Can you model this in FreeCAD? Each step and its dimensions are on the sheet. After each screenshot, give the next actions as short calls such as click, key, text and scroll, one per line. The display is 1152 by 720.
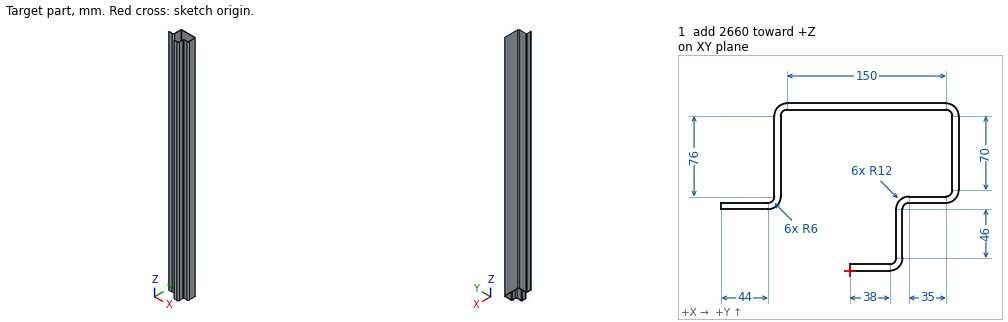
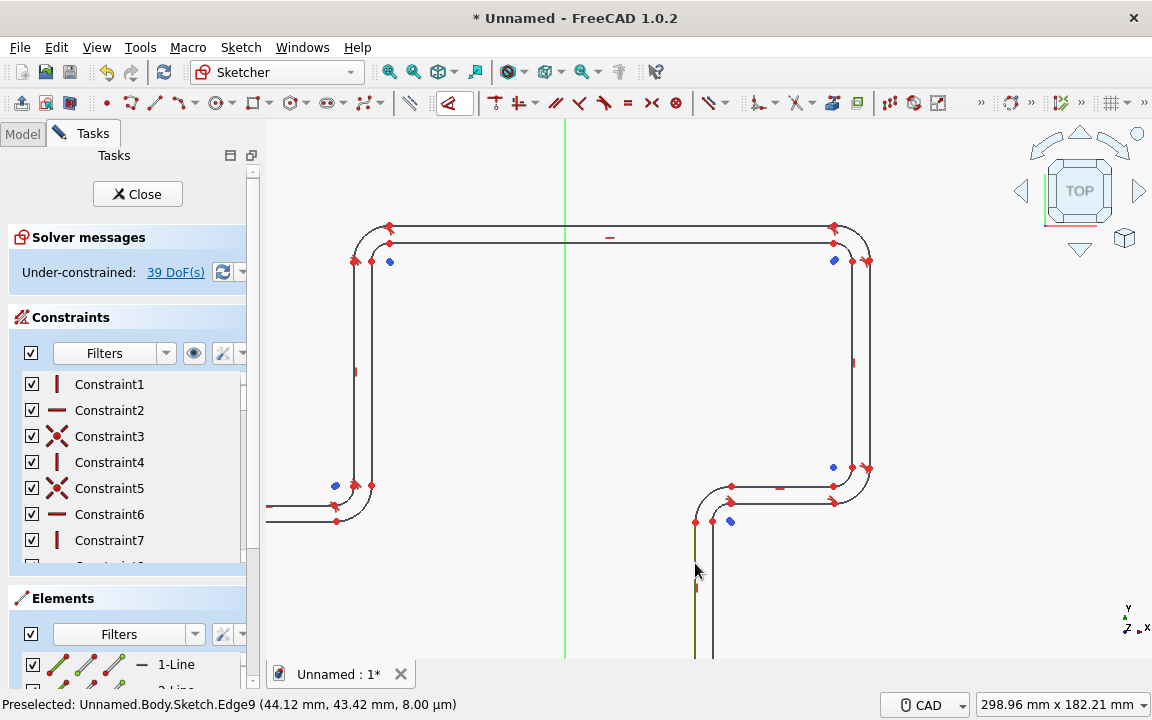
click(715, 491)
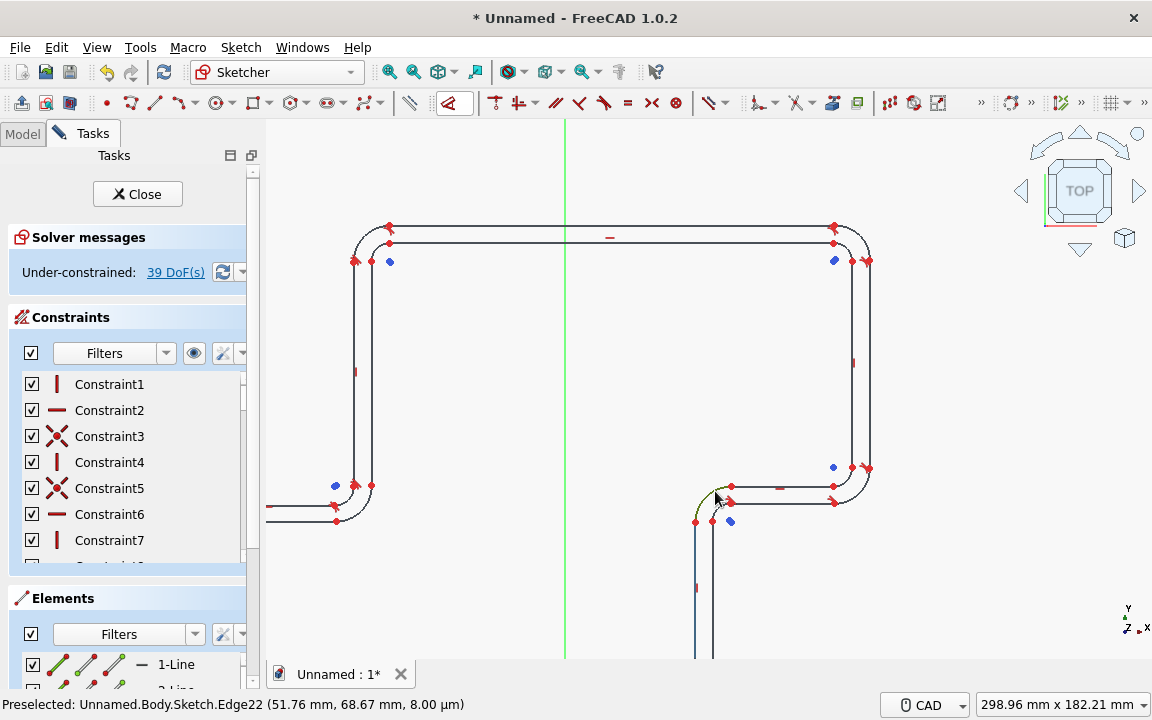
key(t)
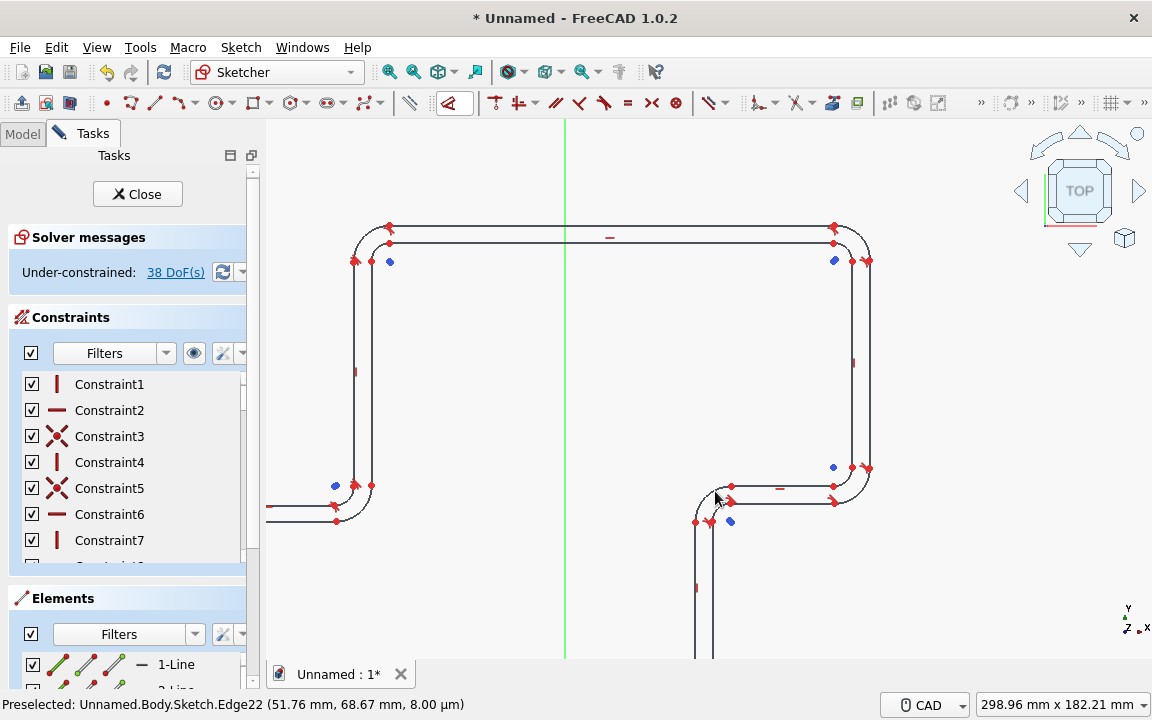
click(695, 563)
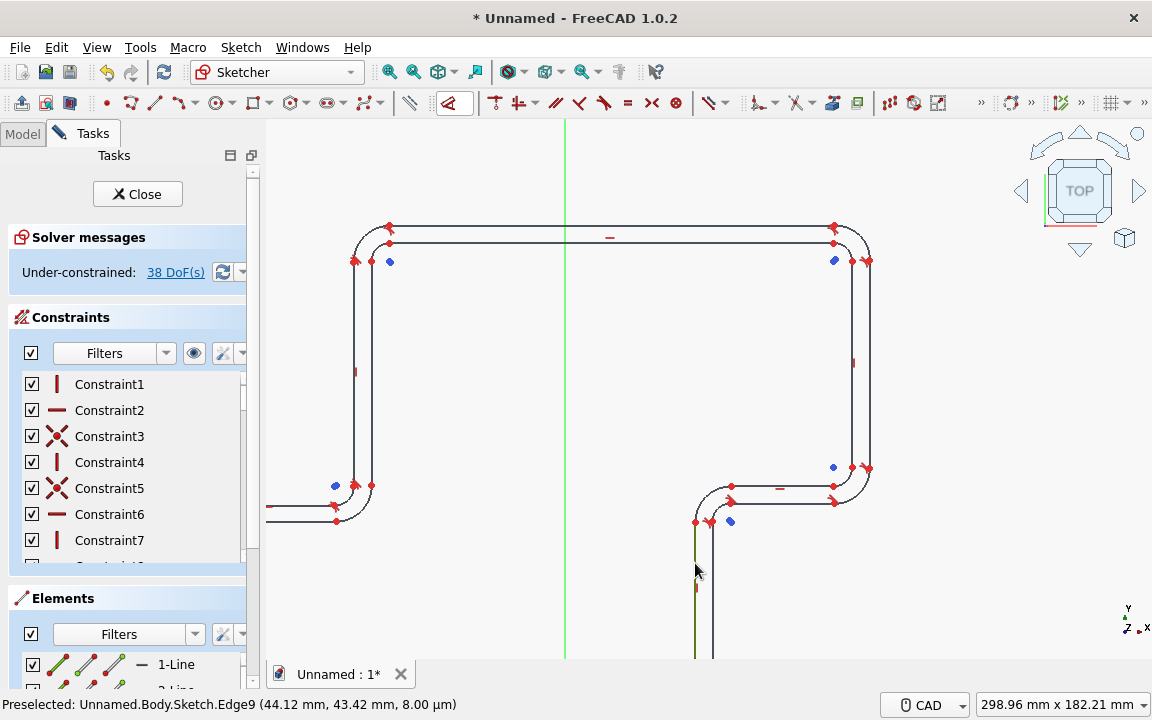
scroll(849, 248, down, 2)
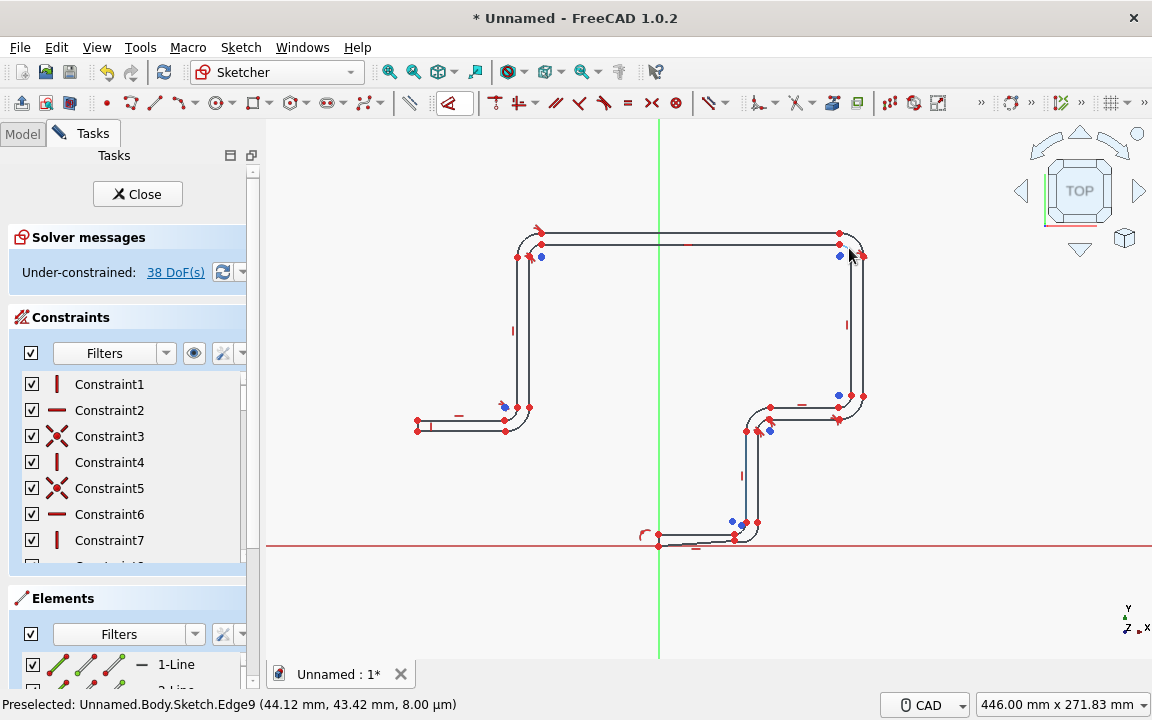
scroll(742, 531, up, 3)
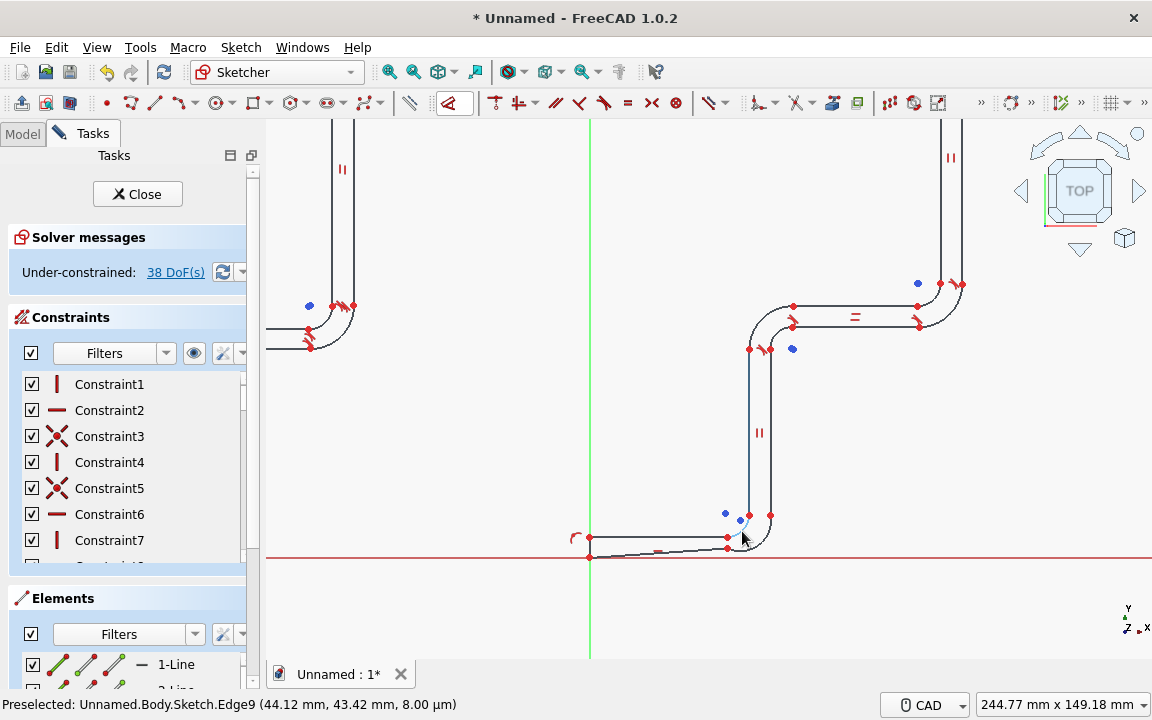
click(742, 530)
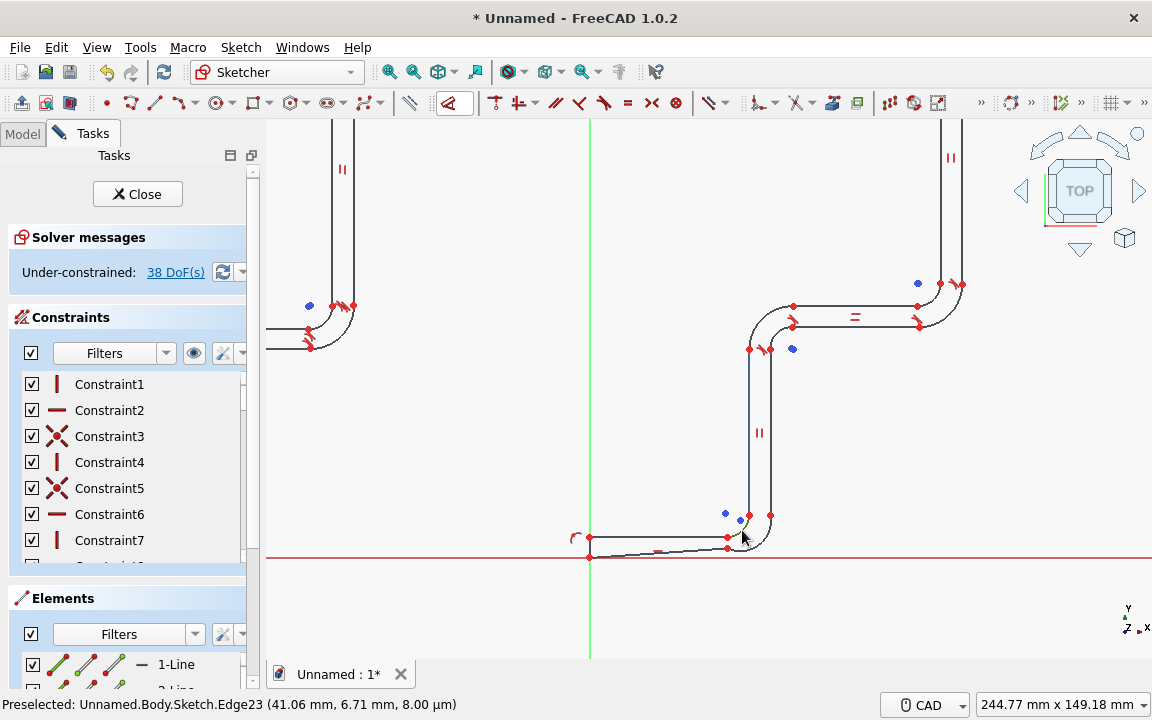
click(604, 104)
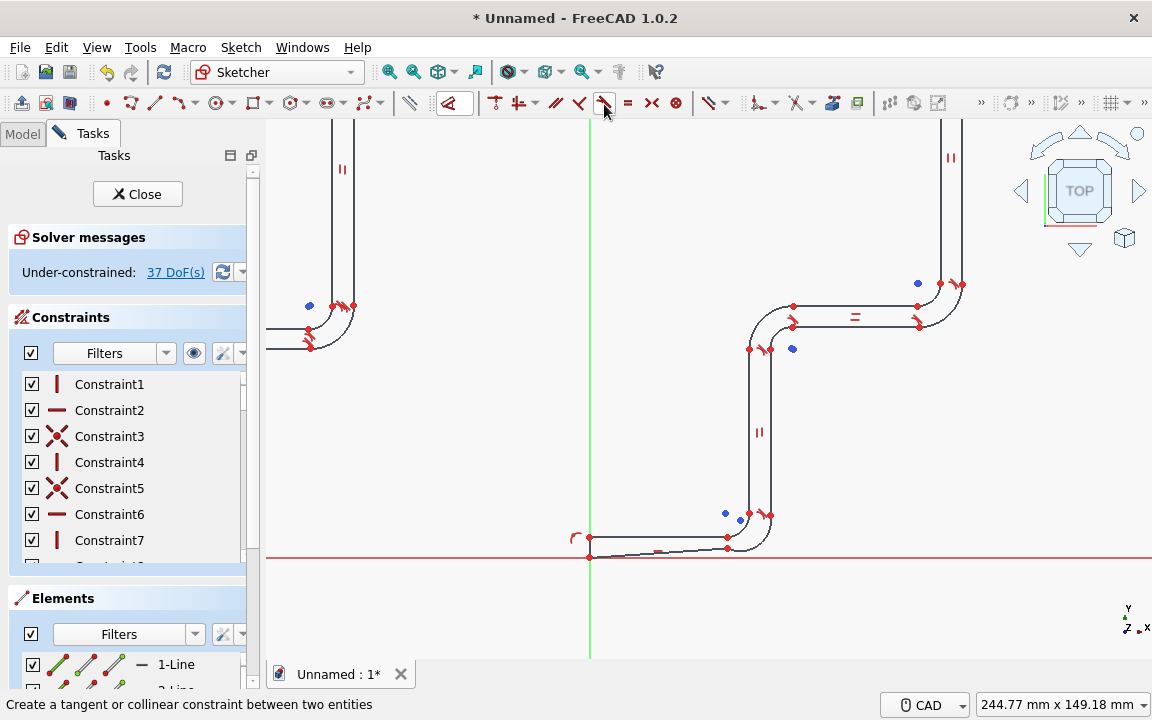
click(686, 537)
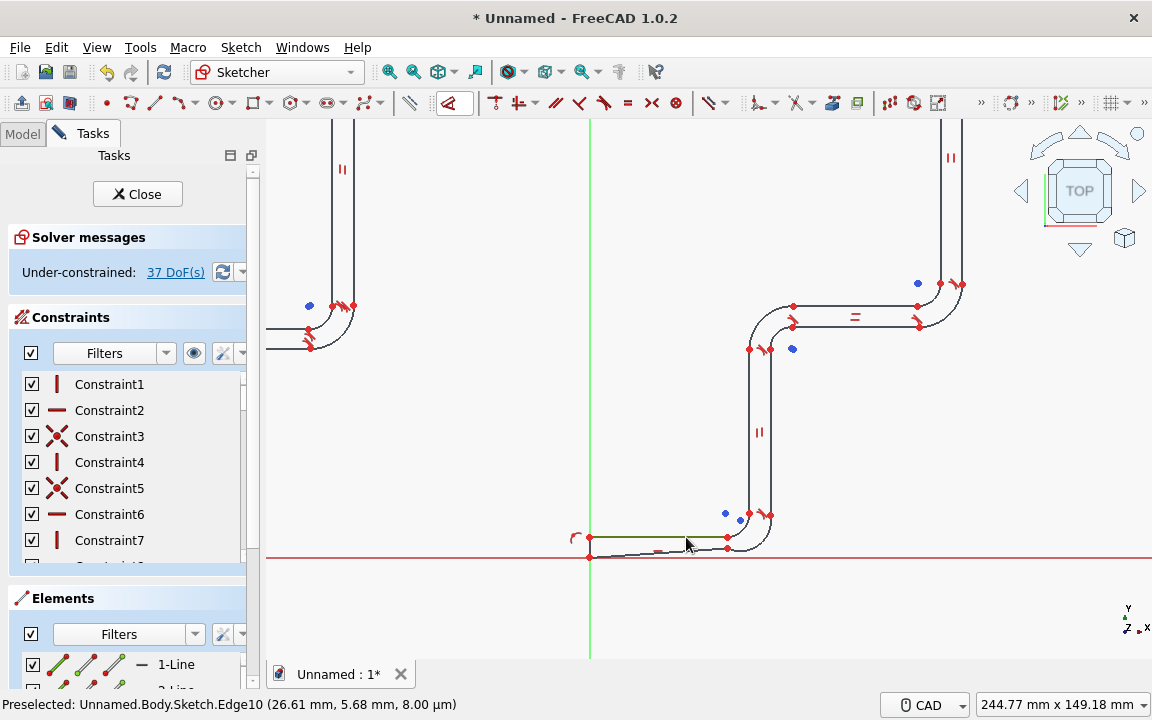
scroll(738, 534, up, 2)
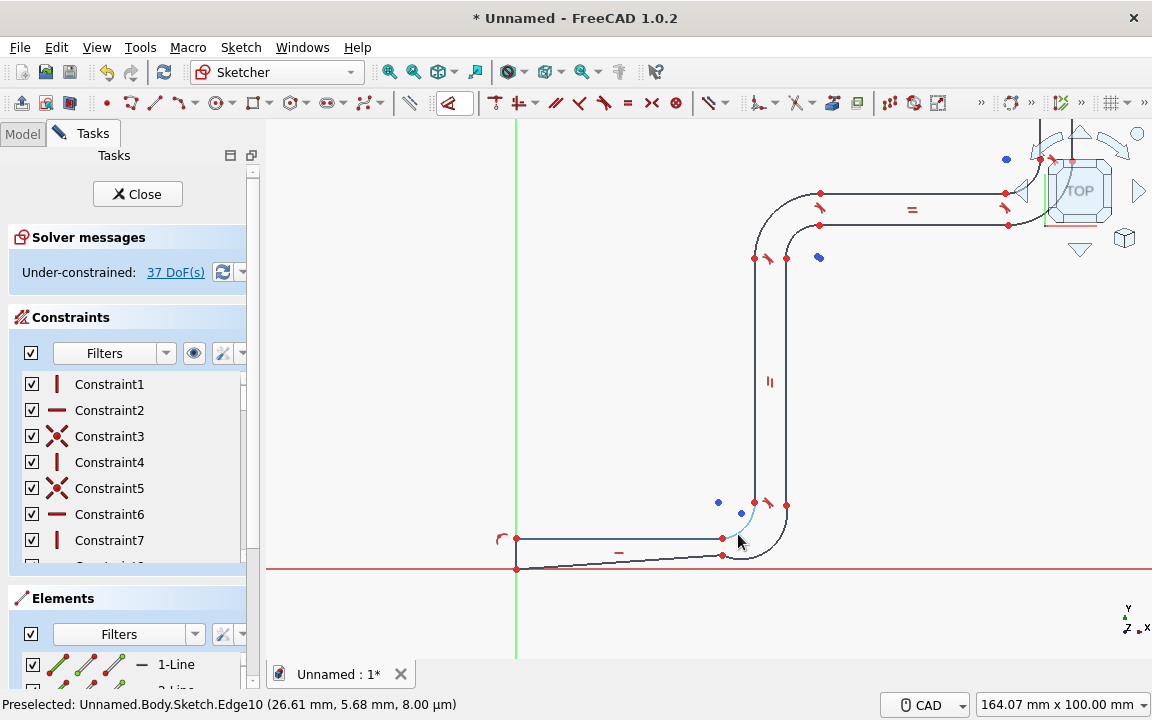
click(737, 534)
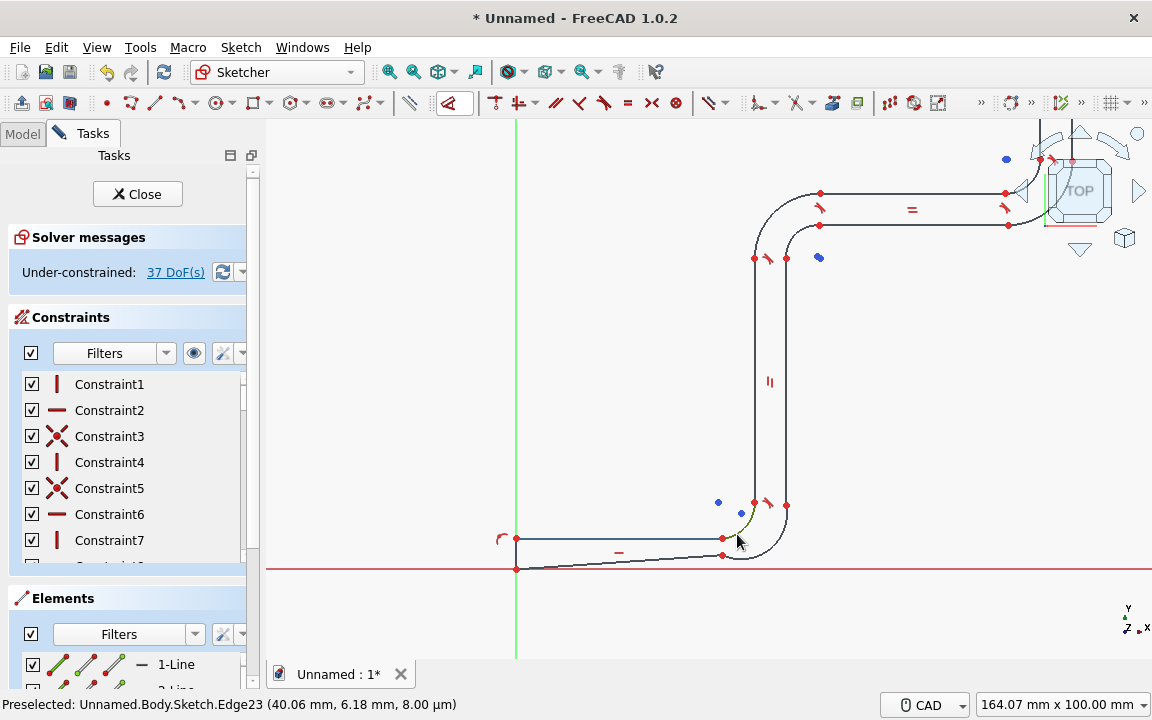
key(t)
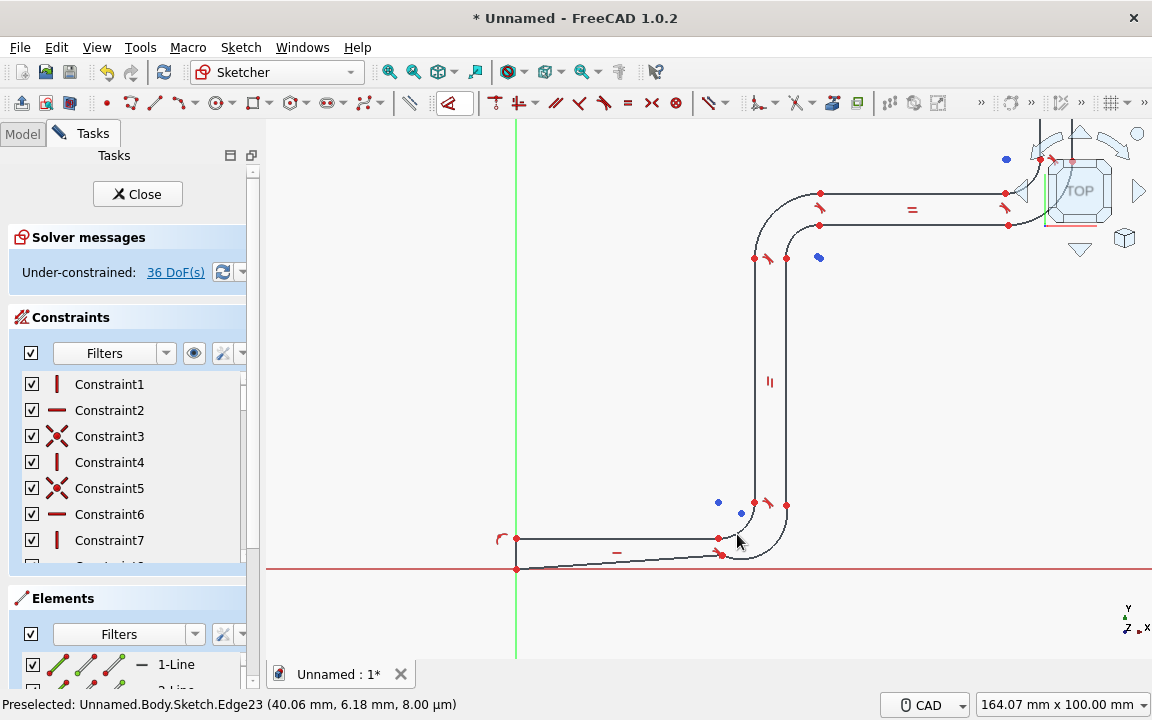
scroll(661, 559, up, 2)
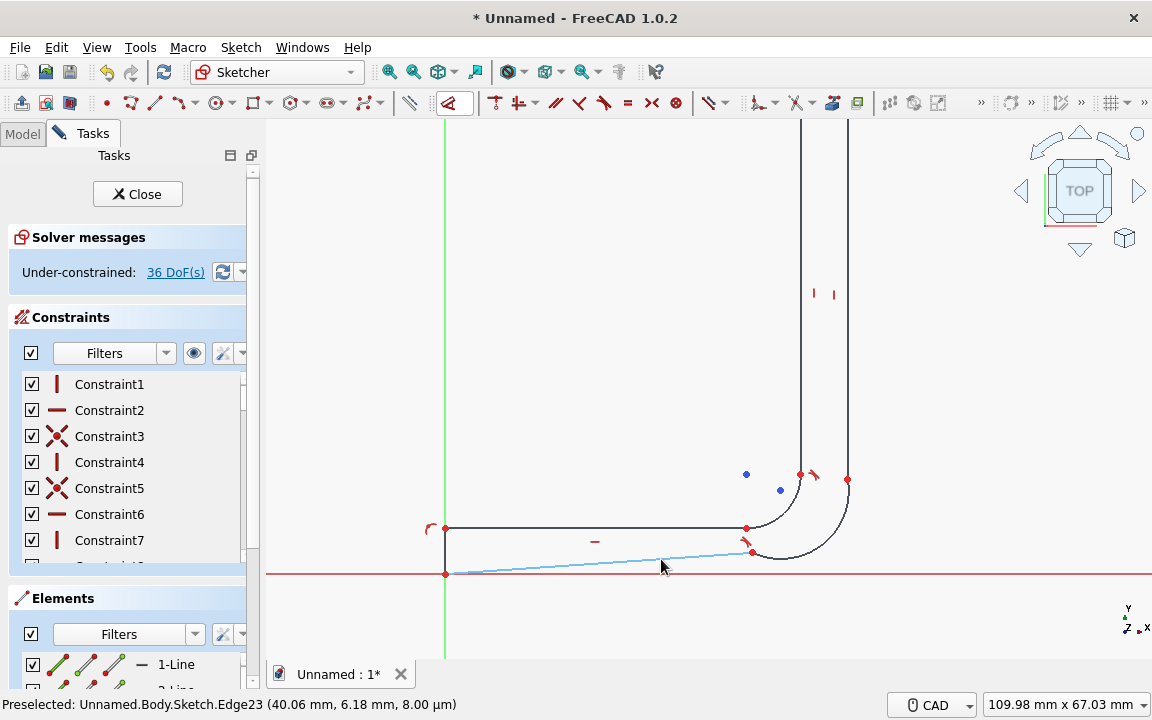
click(660, 559)